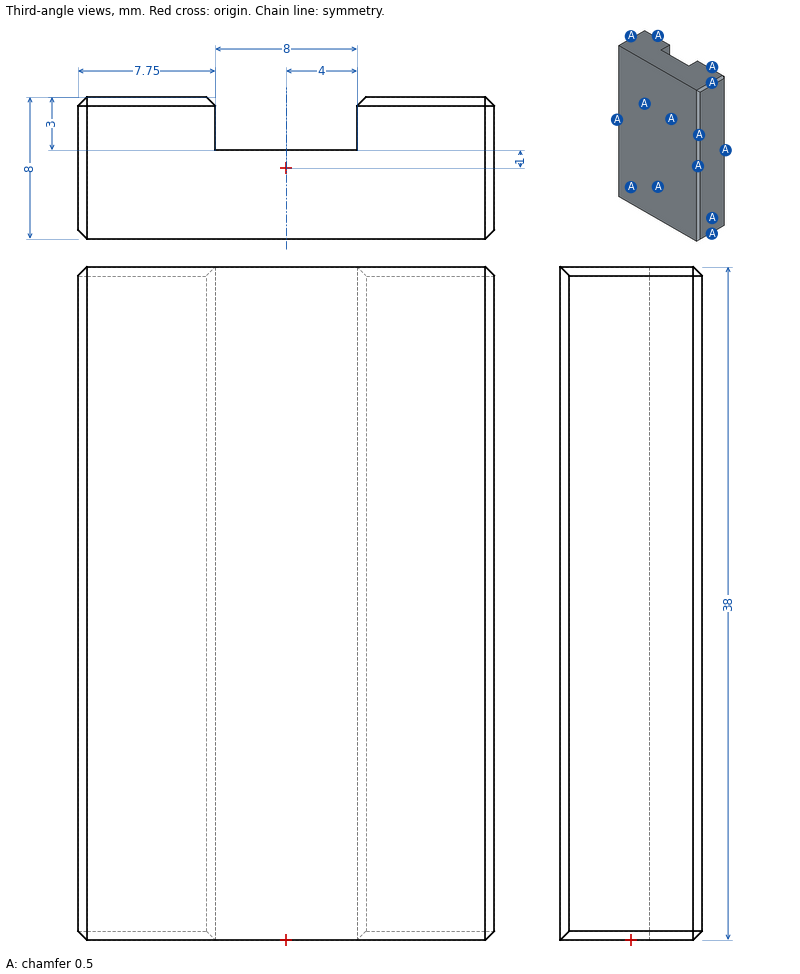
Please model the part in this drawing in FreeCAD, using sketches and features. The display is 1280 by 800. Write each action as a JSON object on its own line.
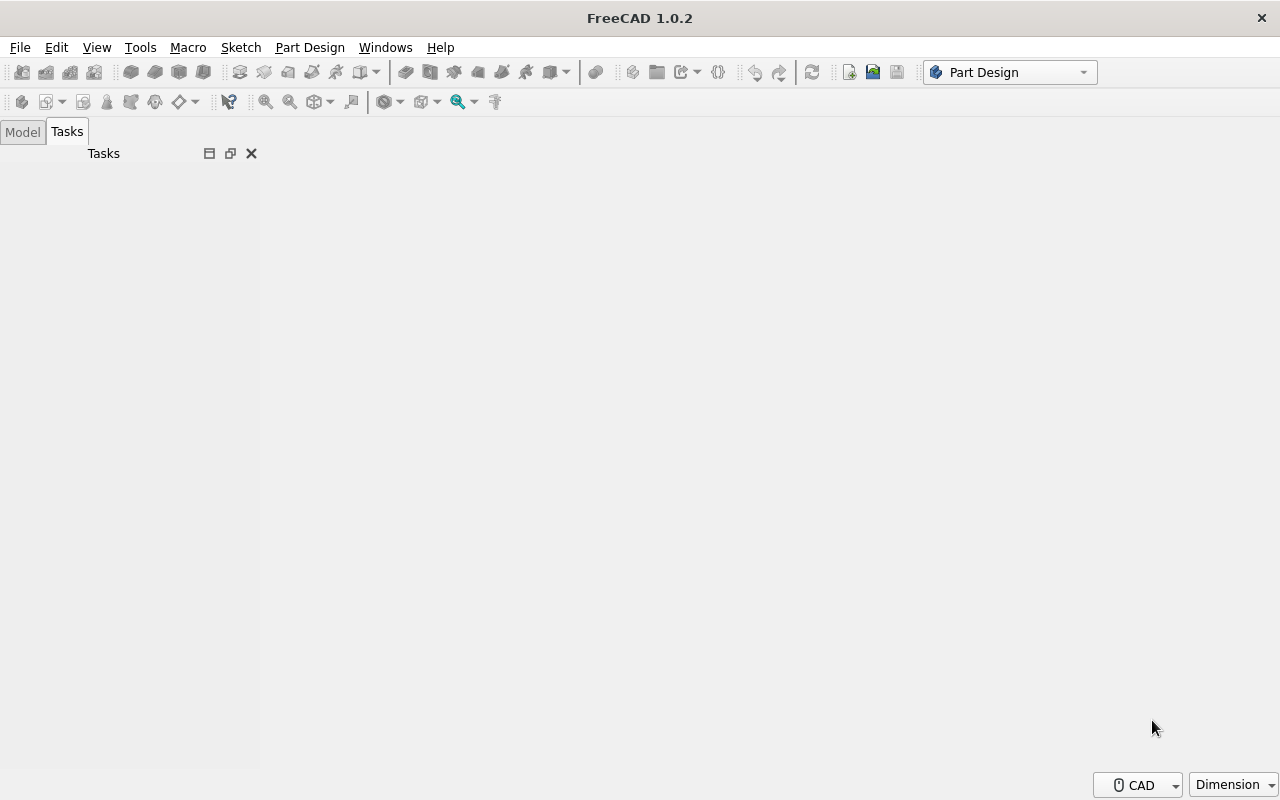
{"action": "left_click", "coordinate": [850, 72]}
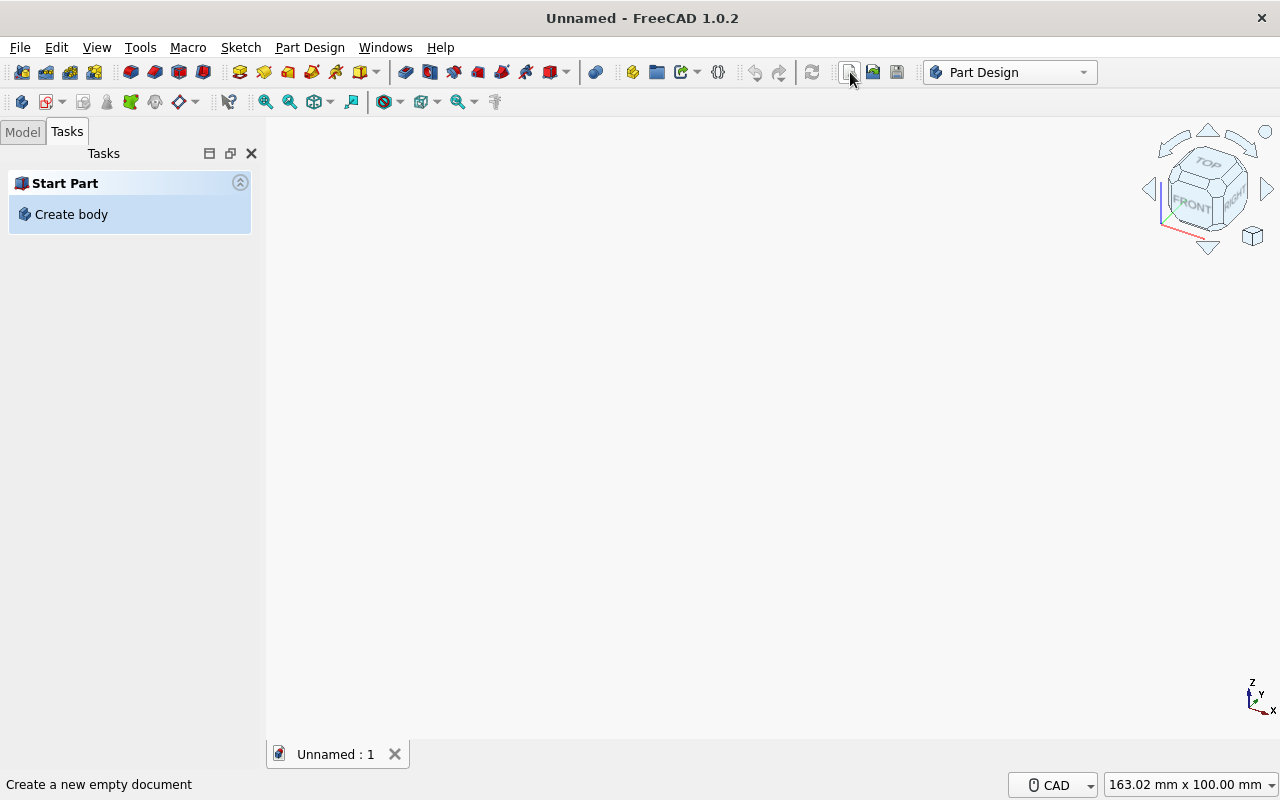
{"action": "left_click", "coordinate": [46, 102]}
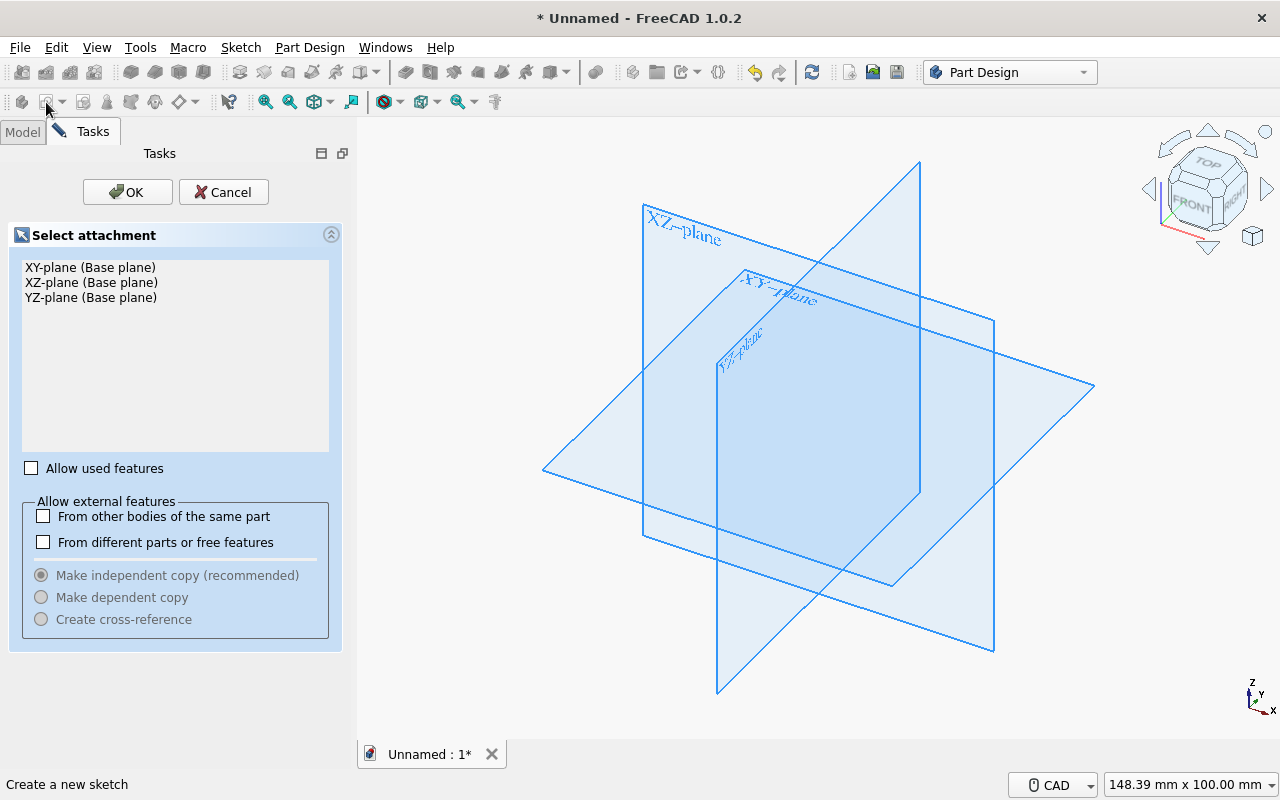
{"action": "left_click", "coordinate": [82, 268]}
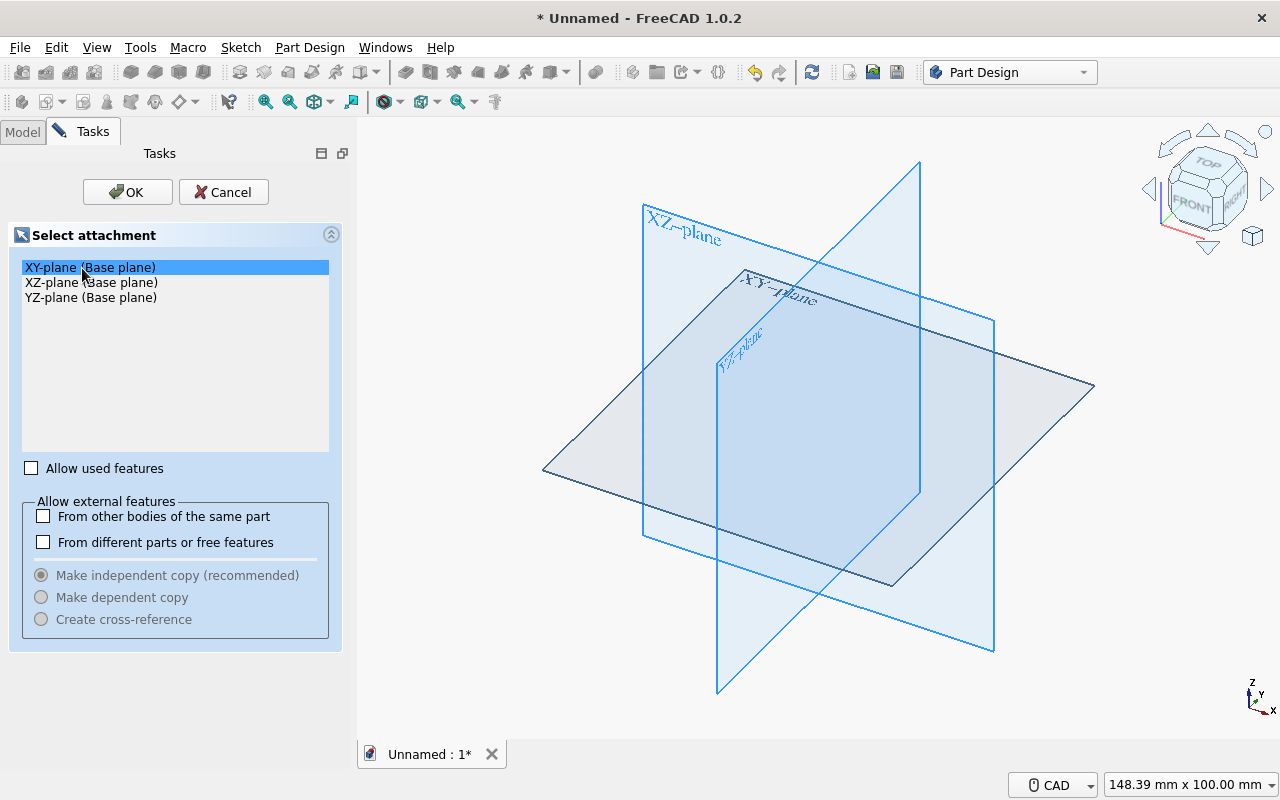
{"action": "left_click", "coordinate": [128, 192]}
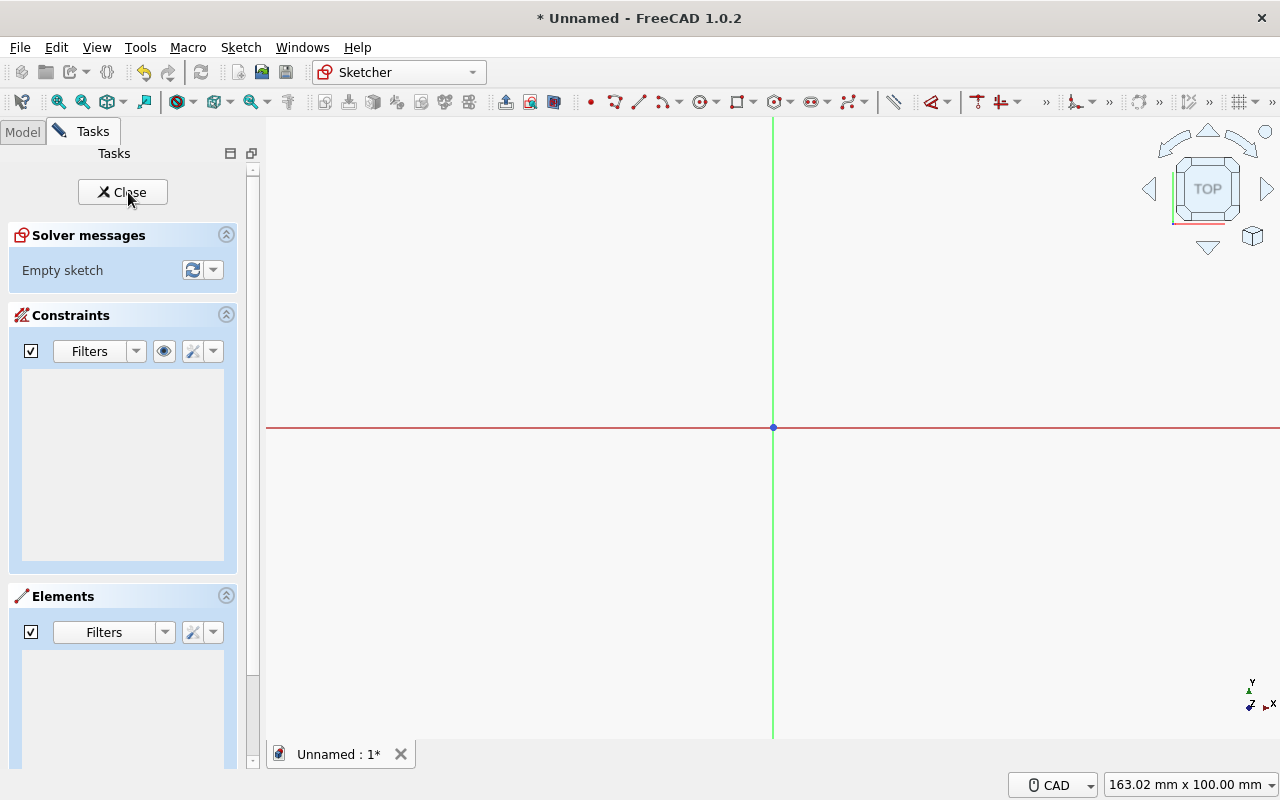
{"action": "scroll", "coordinate": [795, 428], "scroll_direction": "up", "scroll_amount": 7}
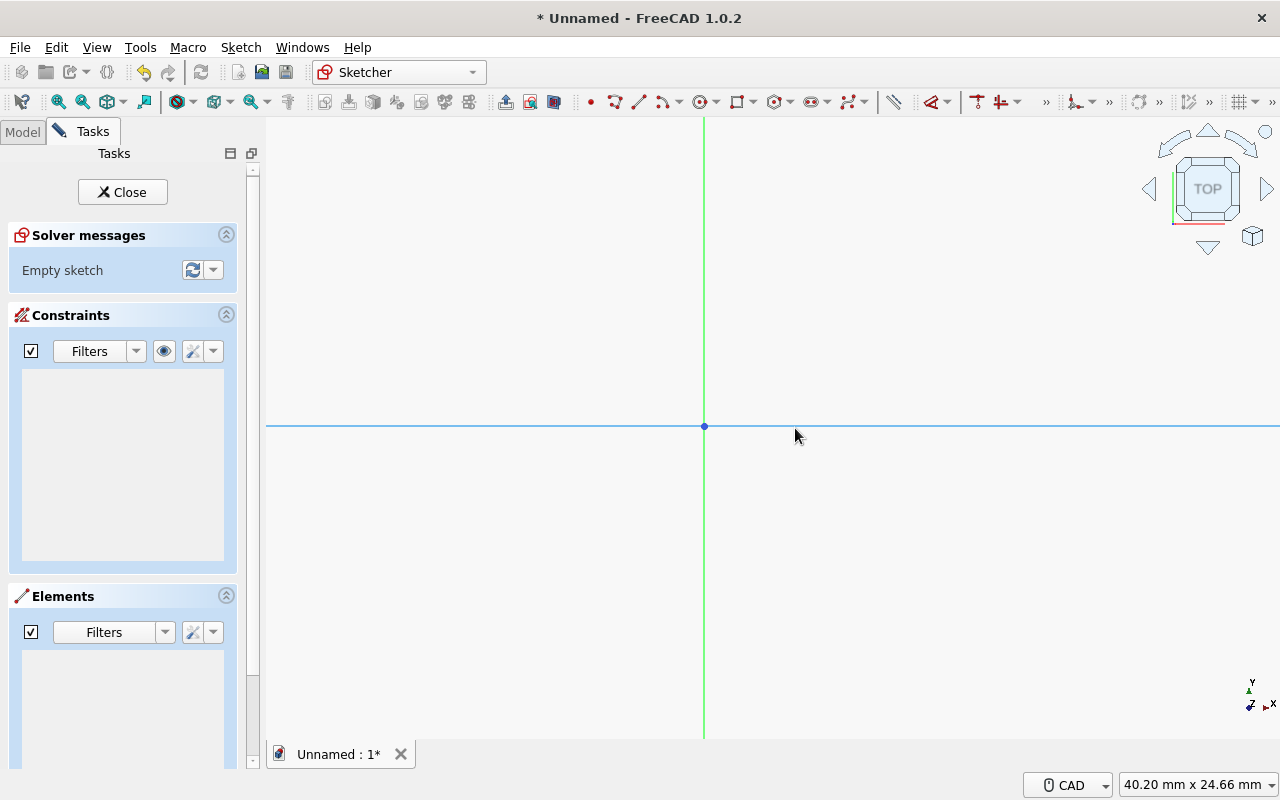
{"action": "key", "text": "g m"}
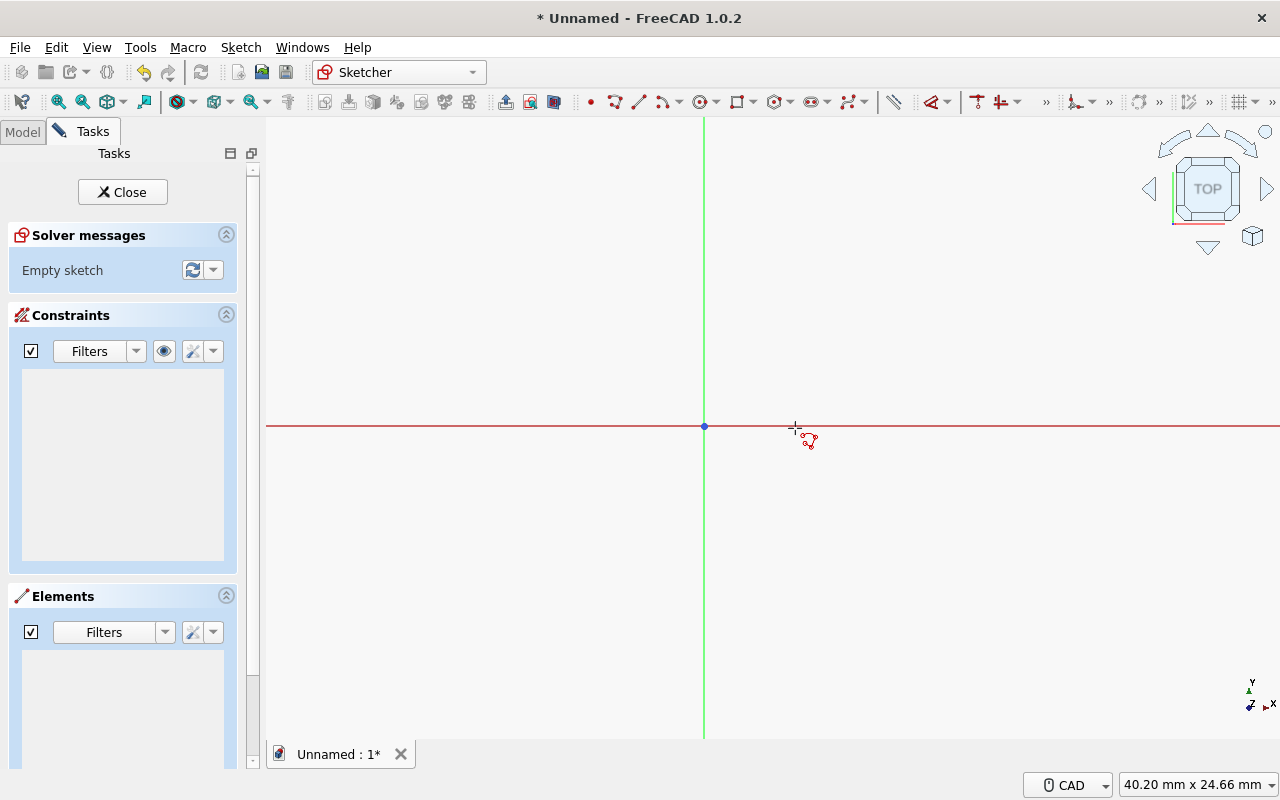
{"action": "left_click", "coordinate": [805, 401]}
{"action": "left_click", "coordinate": [603, 401]}
{"action": "left_click", "coordinate": [603, 326]}
{"action": "left_click", "coordinate": [408, 326]}
{"action": "left_click", "coordinate": [408, 527]}
{"action": "left_click", "coordinate": [1001, 527]}
{"action": "left_click", "coordinate": [1001, 326]}
{"action": "left_click", "coordinate": [805, 326]}
{"action": "left_click", "coordinate": [805, 402]}
{"action": "key", "text": "Escape"}
{"action": "key", "text": "Escape"}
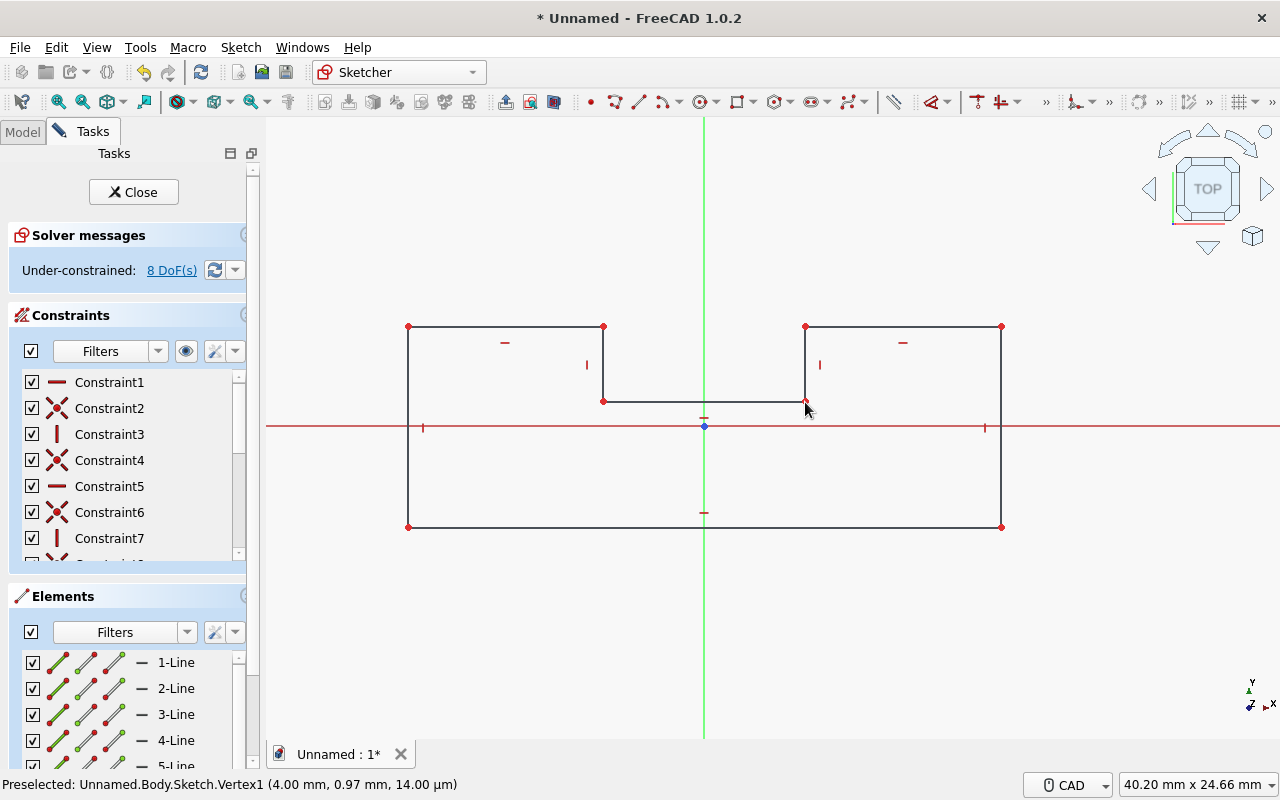
{"action": "left_click", "coordinate": [408, 327]}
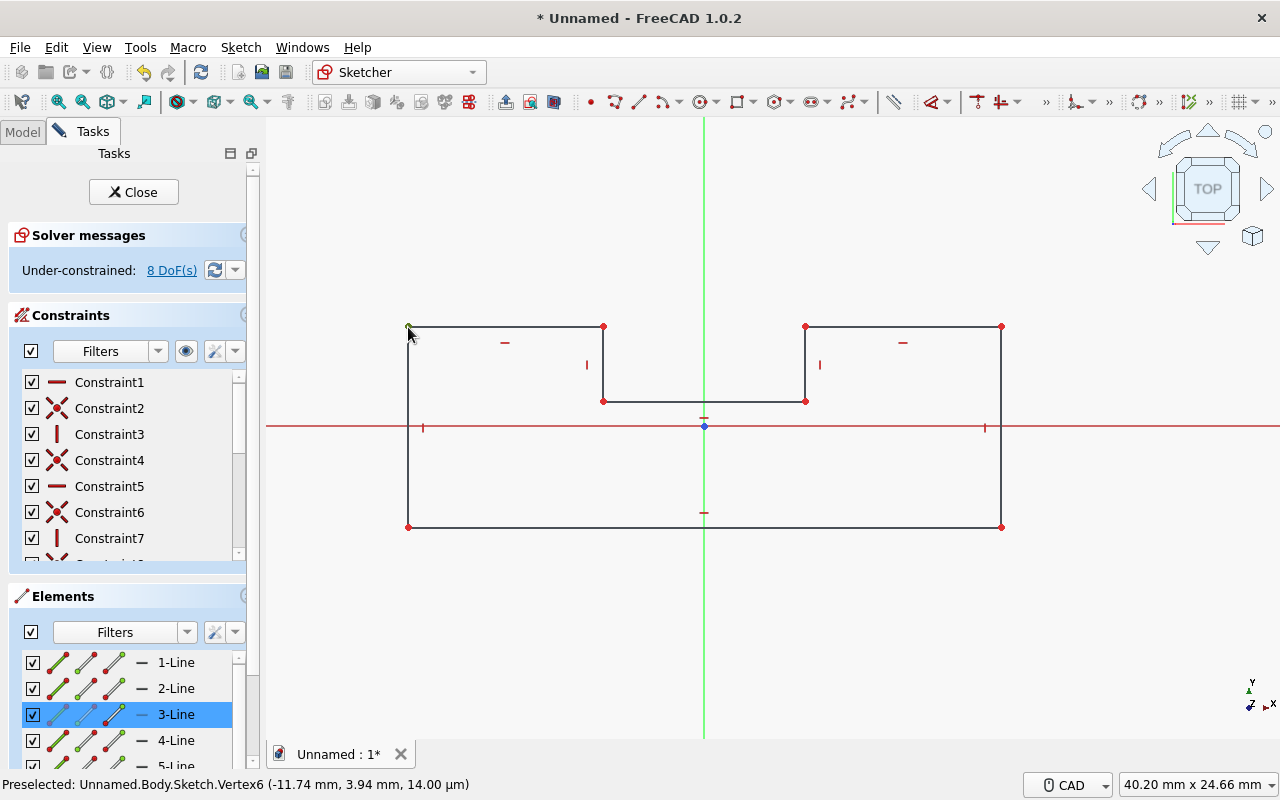
{"action": "left_click", "coordinate": [1001, 327]}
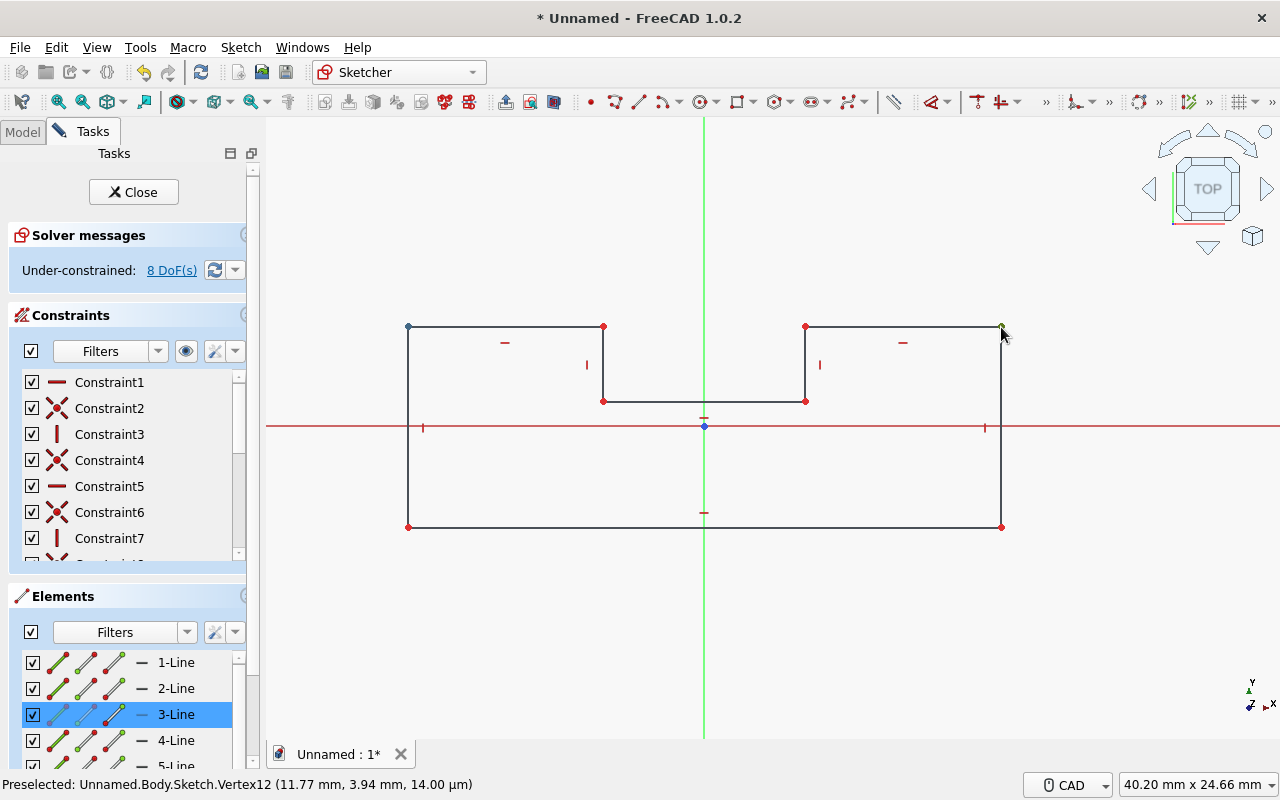
{"action": "left_click", "coordinate": [704, 671]}